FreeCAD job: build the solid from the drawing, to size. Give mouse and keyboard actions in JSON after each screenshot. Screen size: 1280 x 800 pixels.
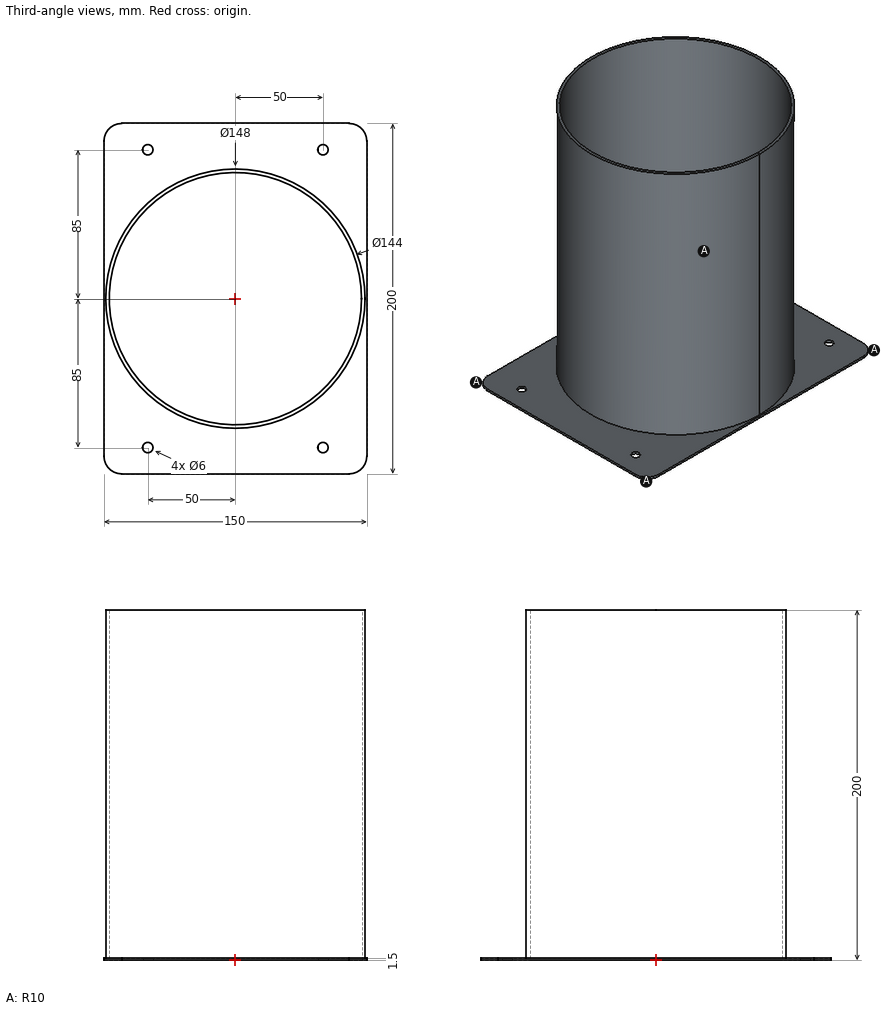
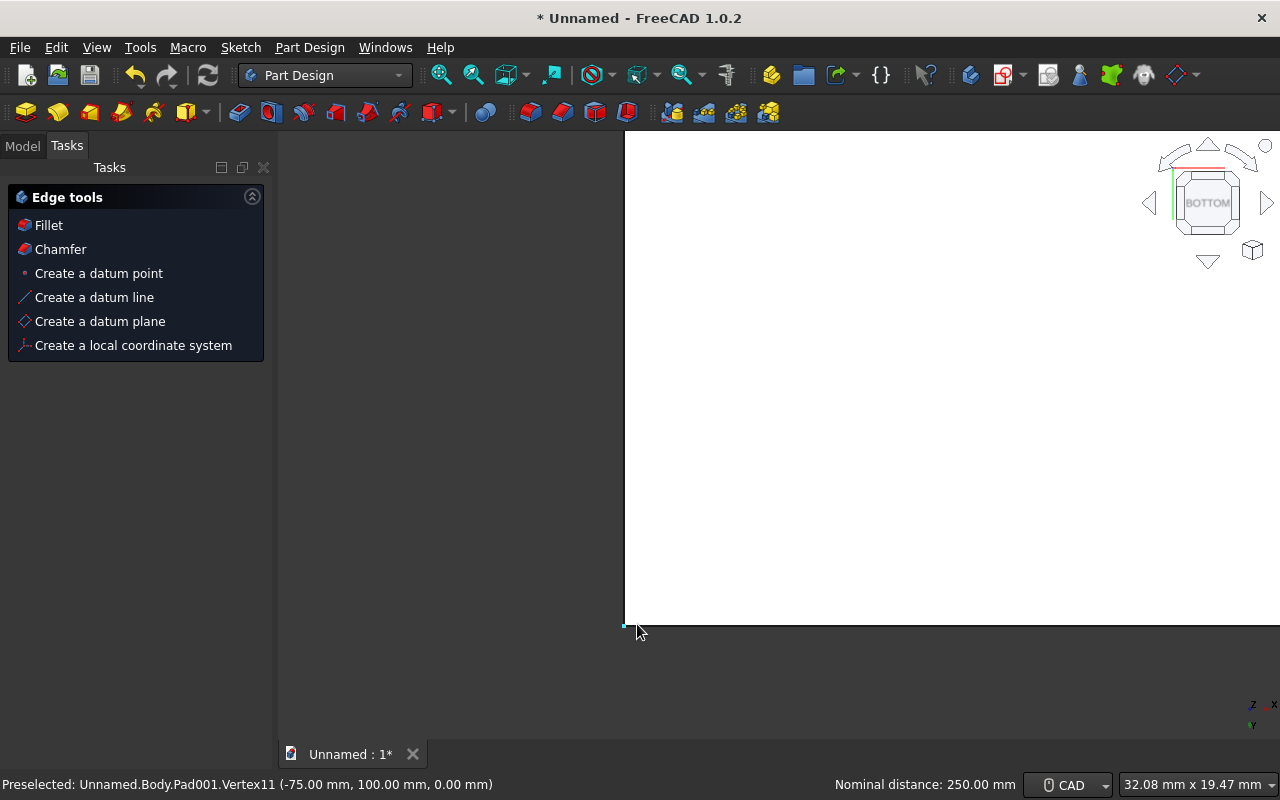
{"action": "left_click", "coordinate": [442, 76]}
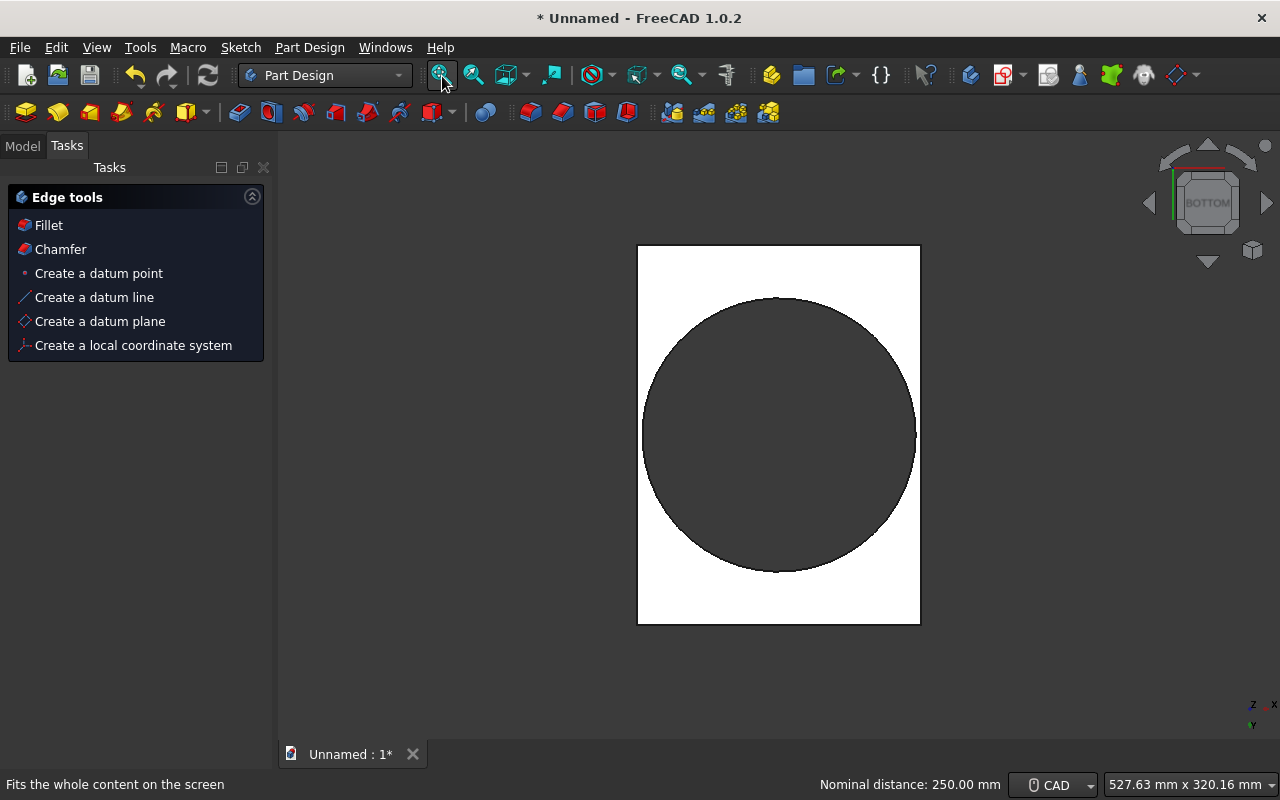
{"action": "key", "text": "4"}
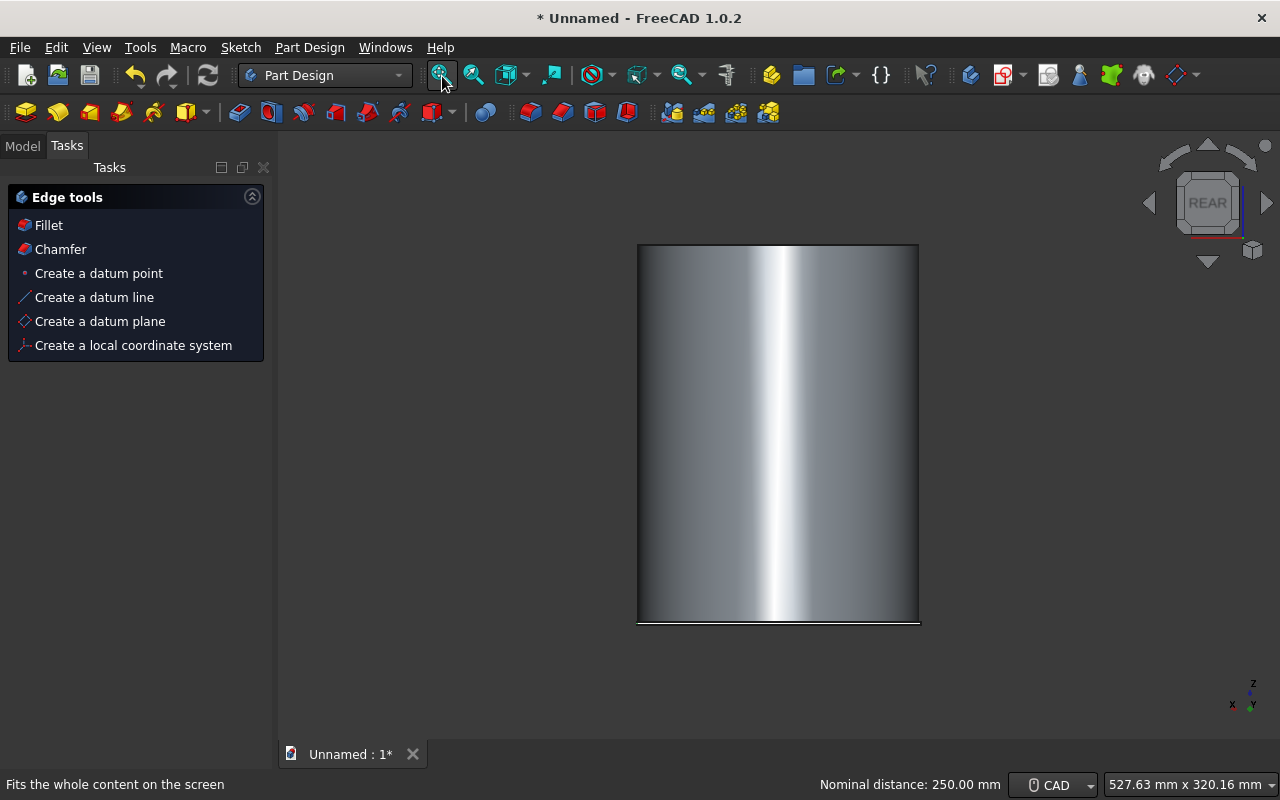
{"action": "scroll", "coordinate": [921, 622], "scroll_direction": "up", "scroll_amount": 14}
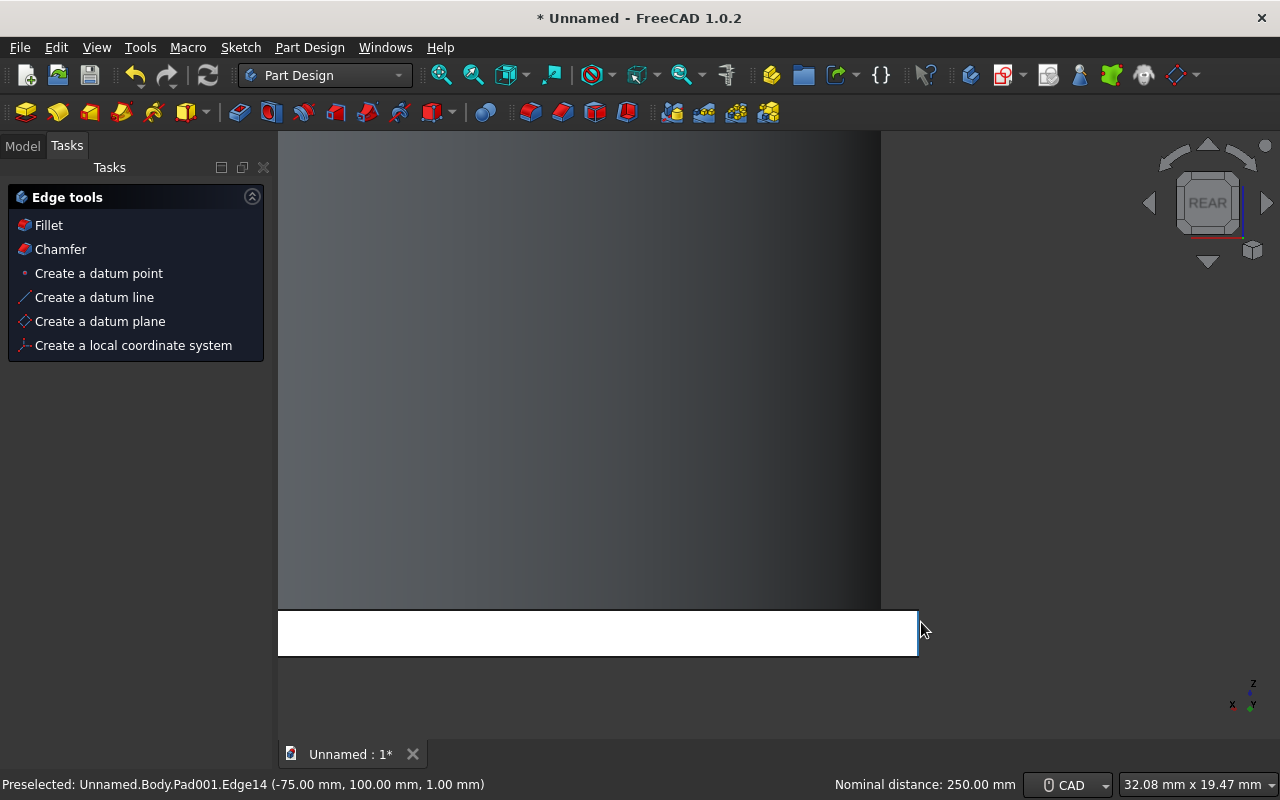
{"action": "left_click", "coordinate": [918, 633], "text": "ctrl"}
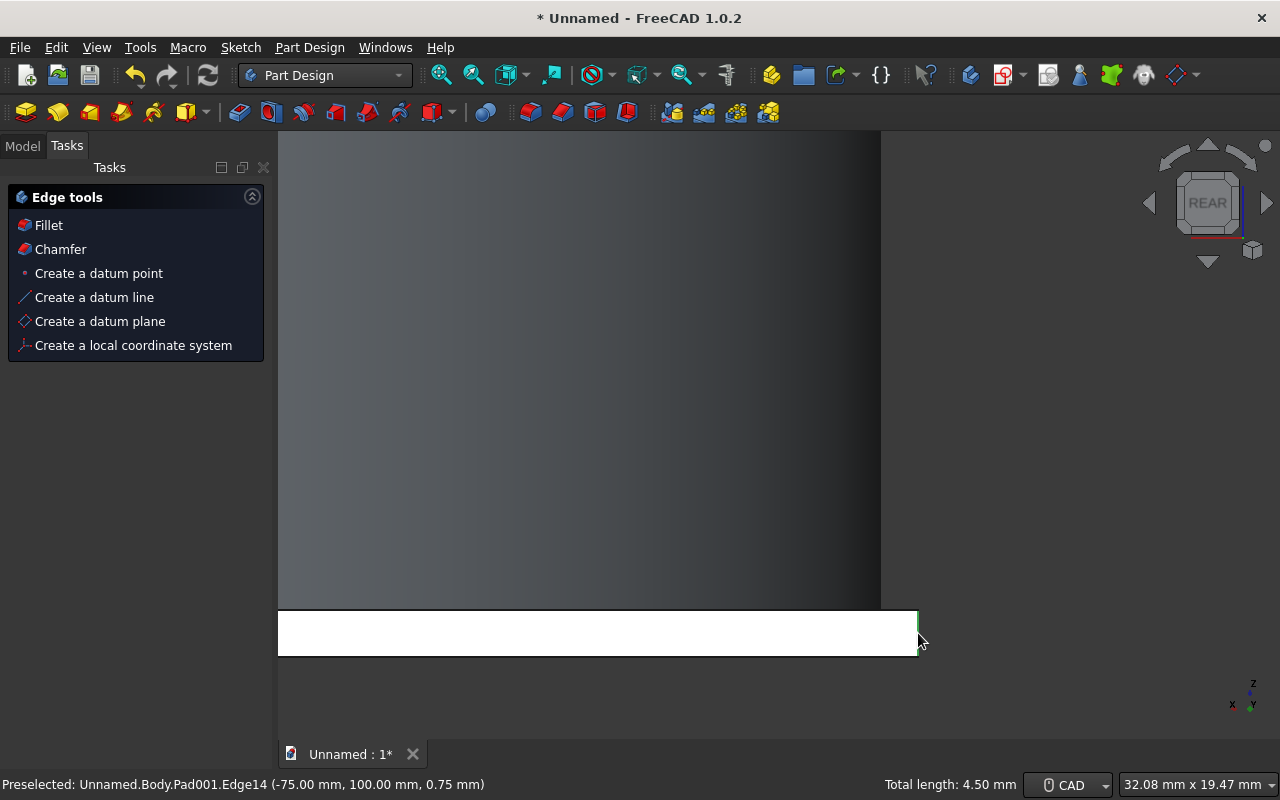
{"action": "left_click", "coordinate": [442, 76]}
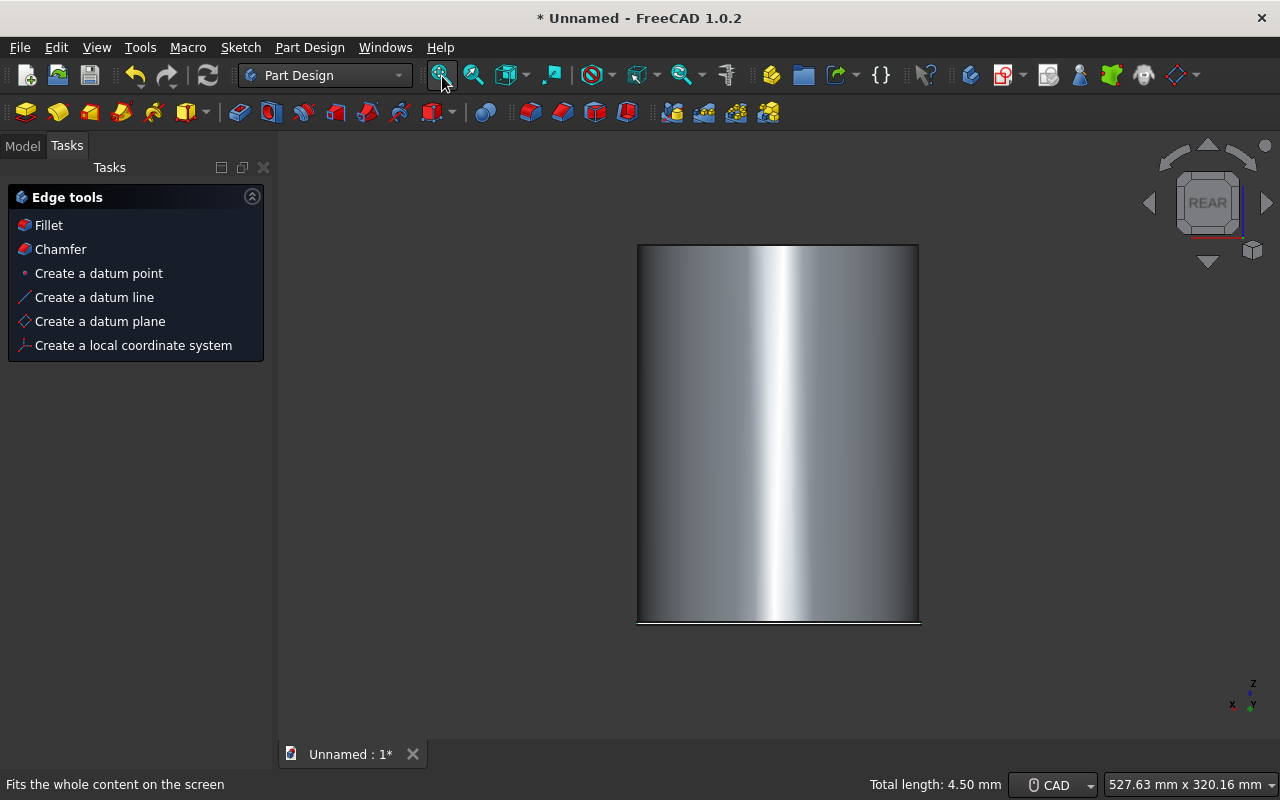
{"action": "key", "text": "6"}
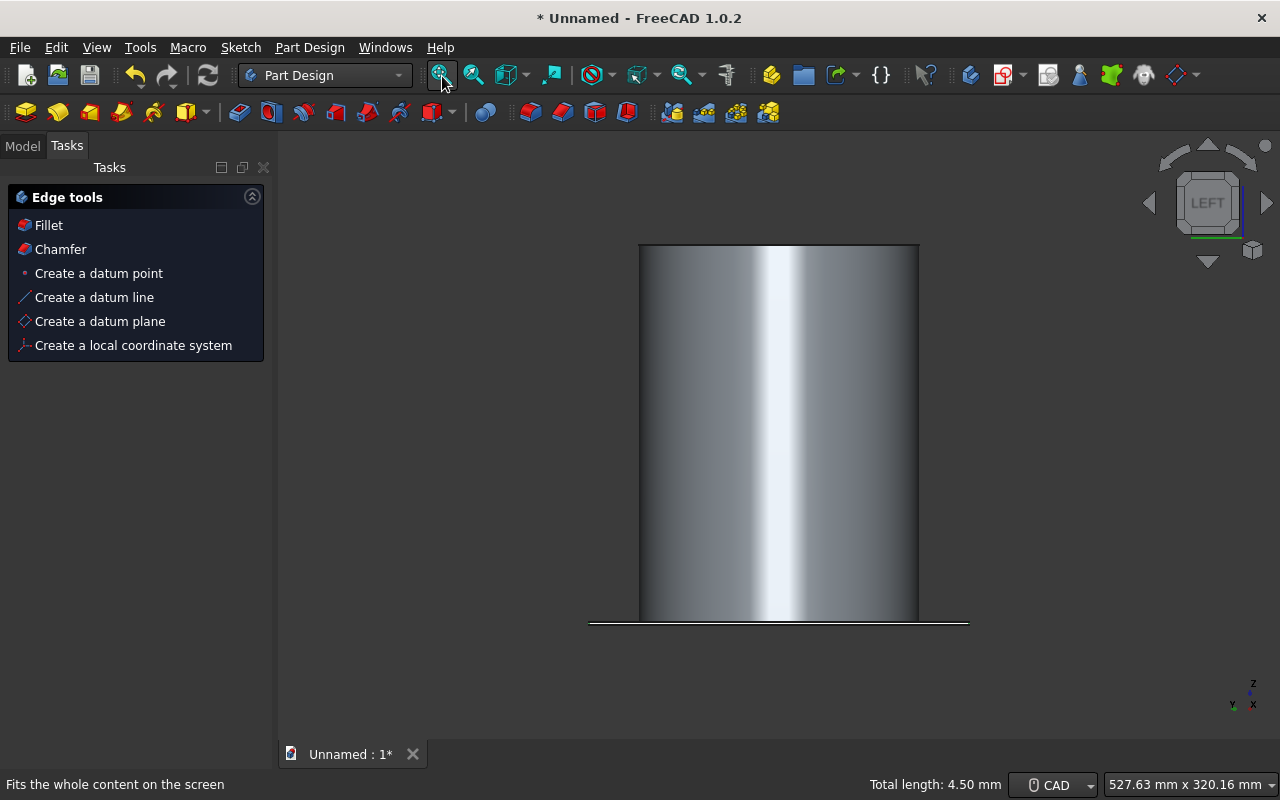
{"action": "scroll", "coordinate": [969, 622], "scroll_direction": "up", "scroll_amount": 14}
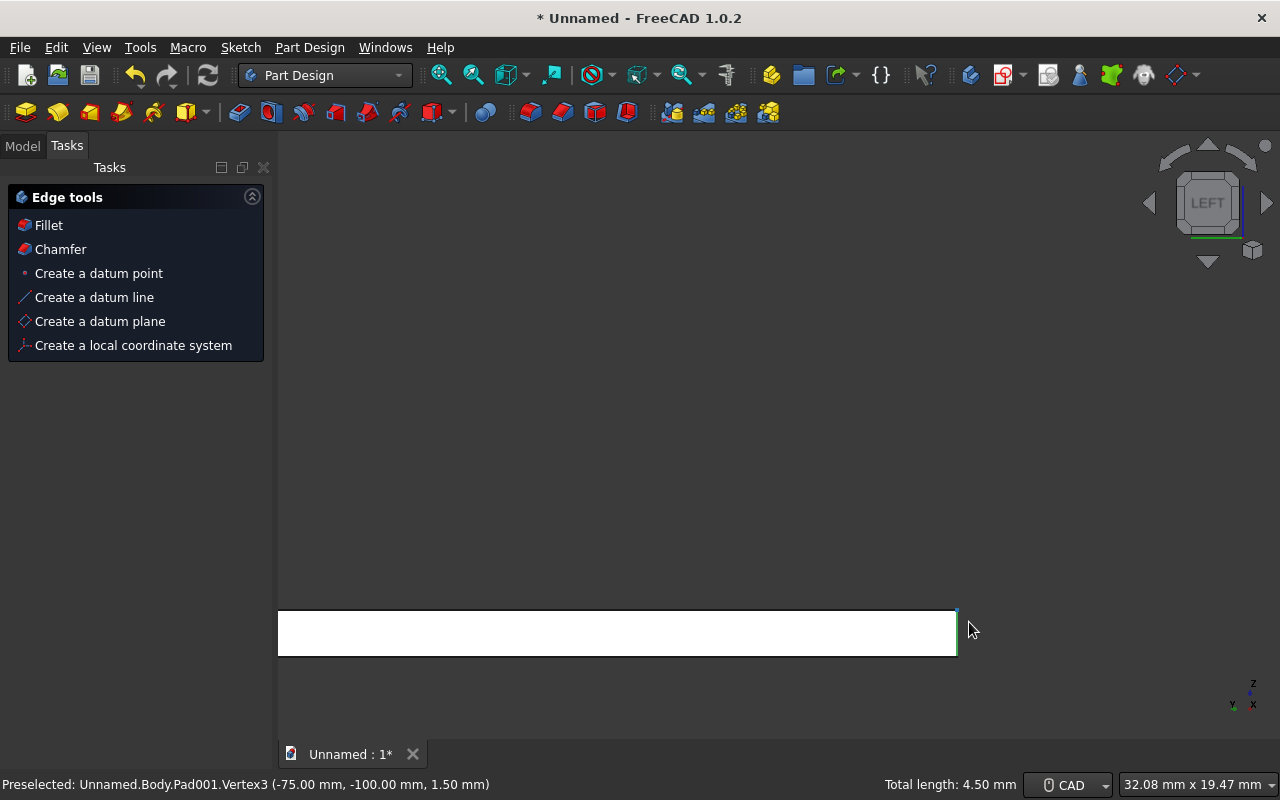
{"action": "left_click", "coordinate": [442, 76]}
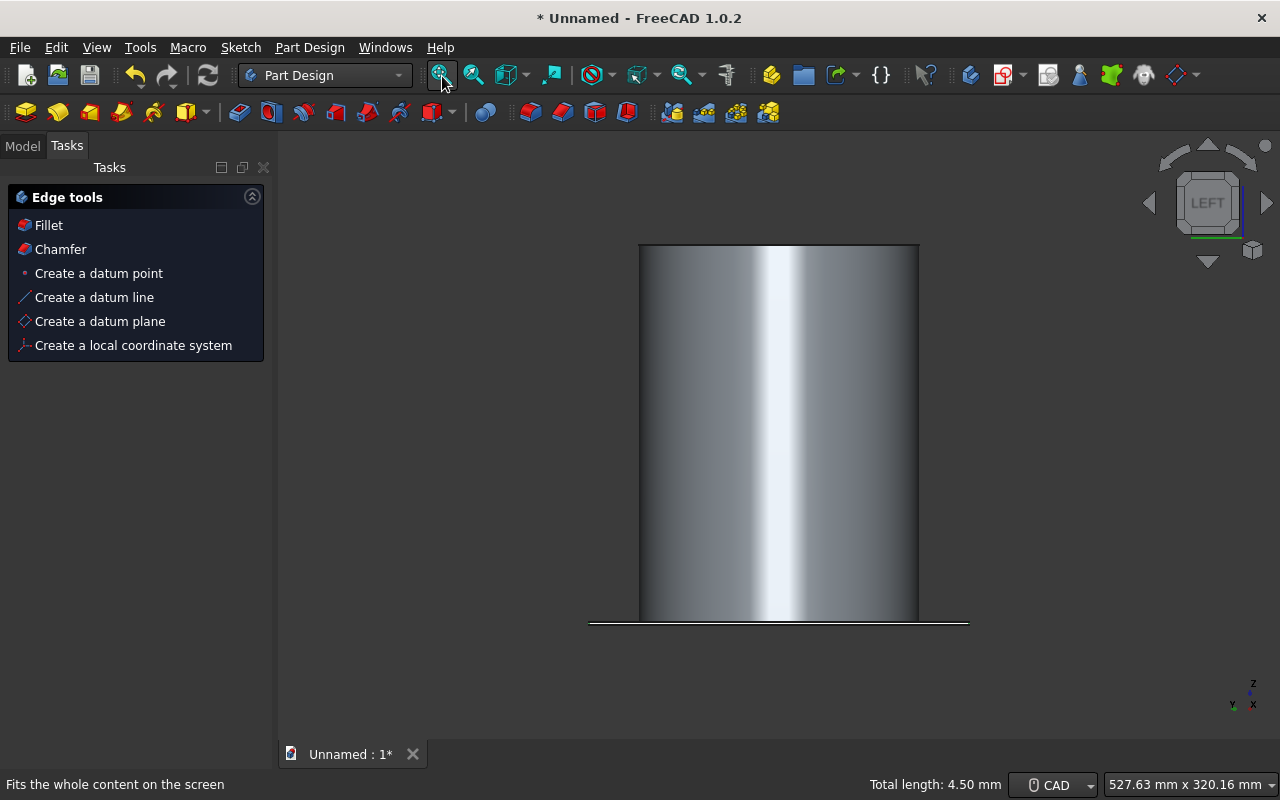
{"action": "key", "text": "v 3"}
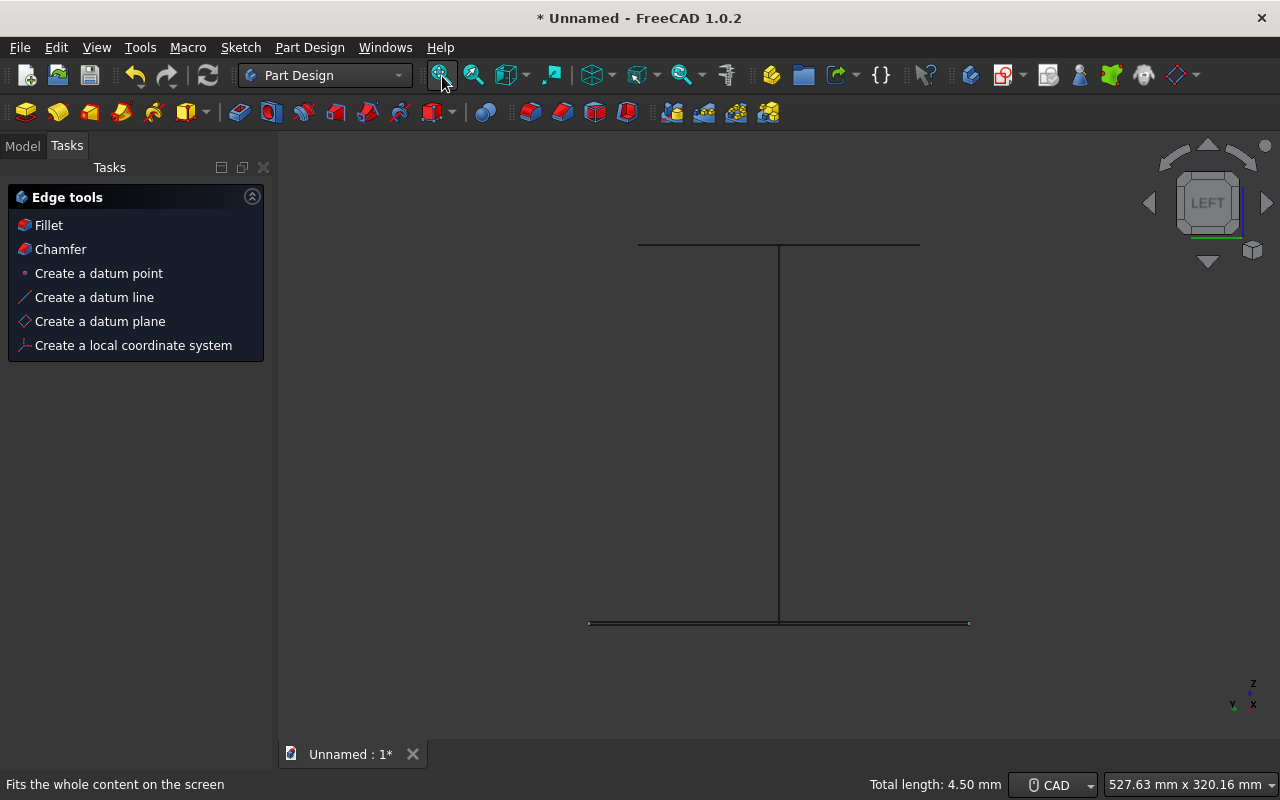
{"action": "key", "text": "0"}